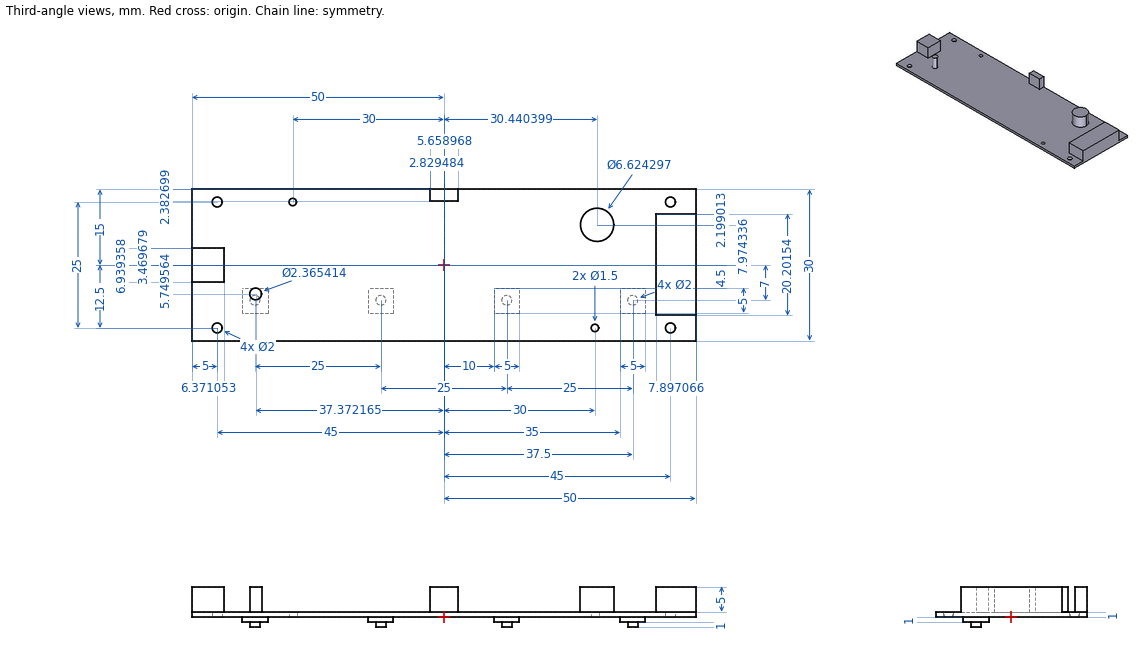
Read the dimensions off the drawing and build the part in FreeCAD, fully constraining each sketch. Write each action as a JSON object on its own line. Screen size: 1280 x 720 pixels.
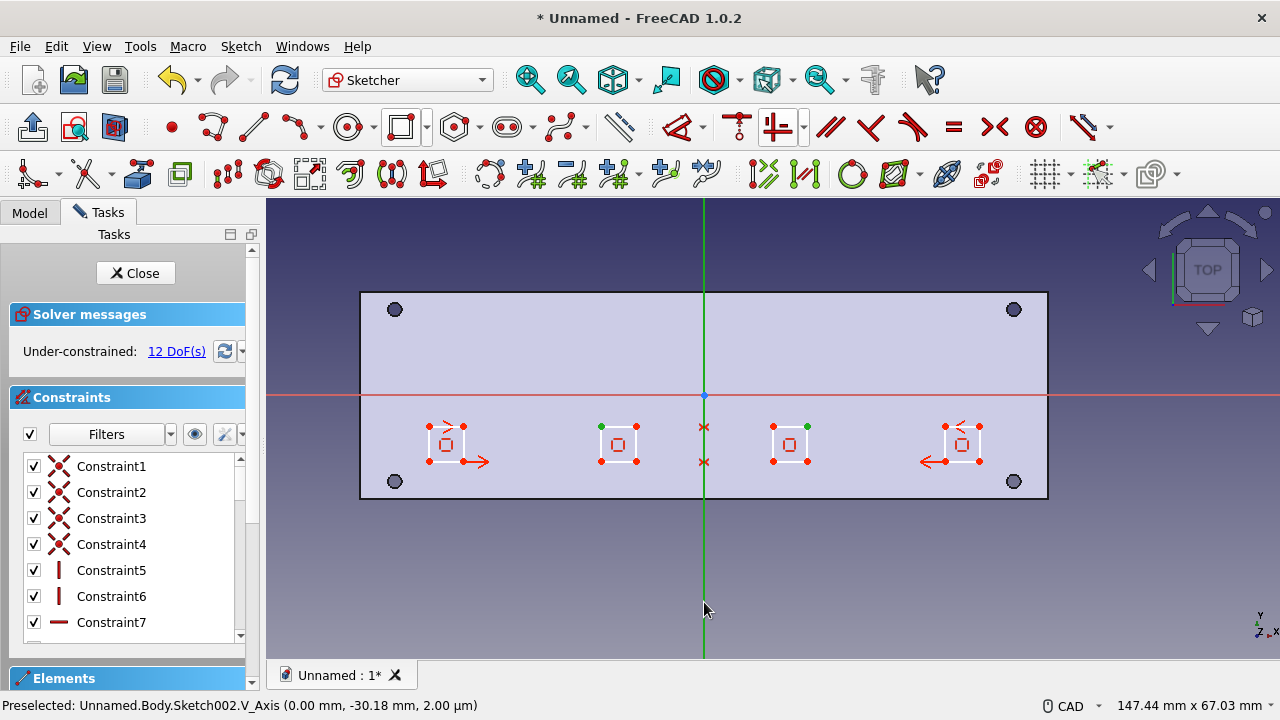
{"action": "key", "text": "s"}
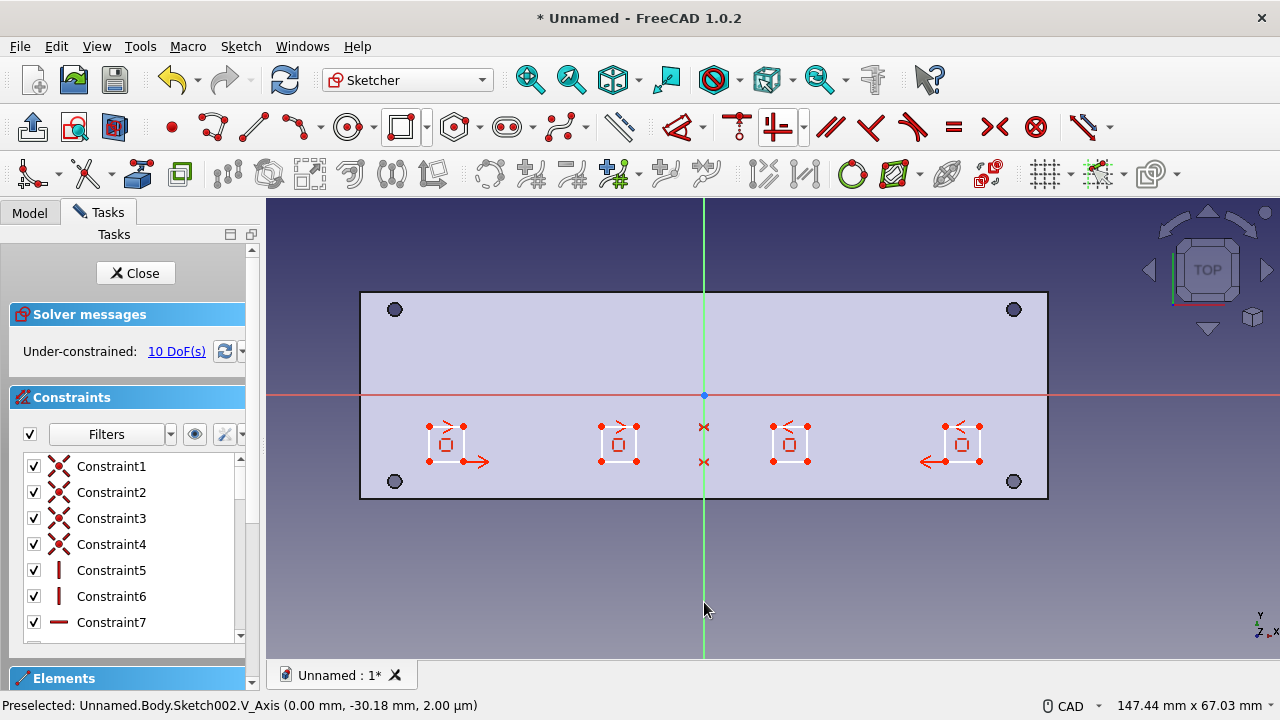
{"action": "left_click", "coordinate": [773, 462]}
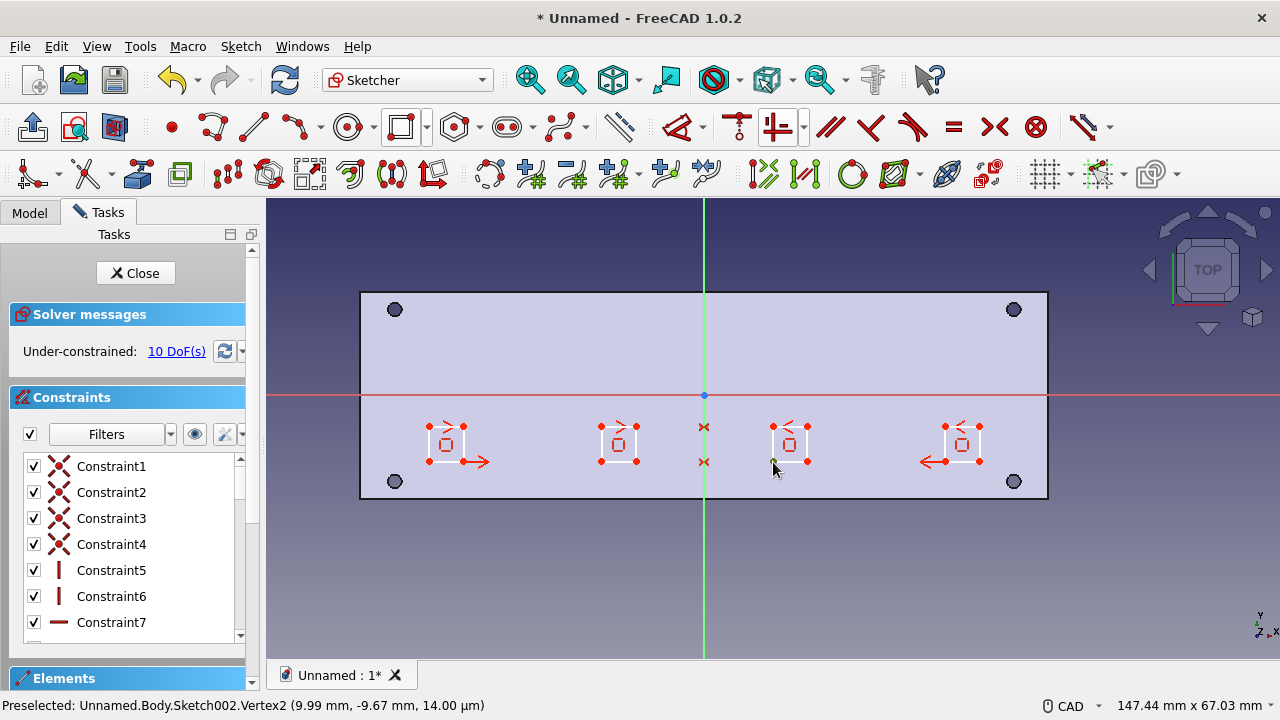
{"action": "left_click", "coordinate": [636, 462]}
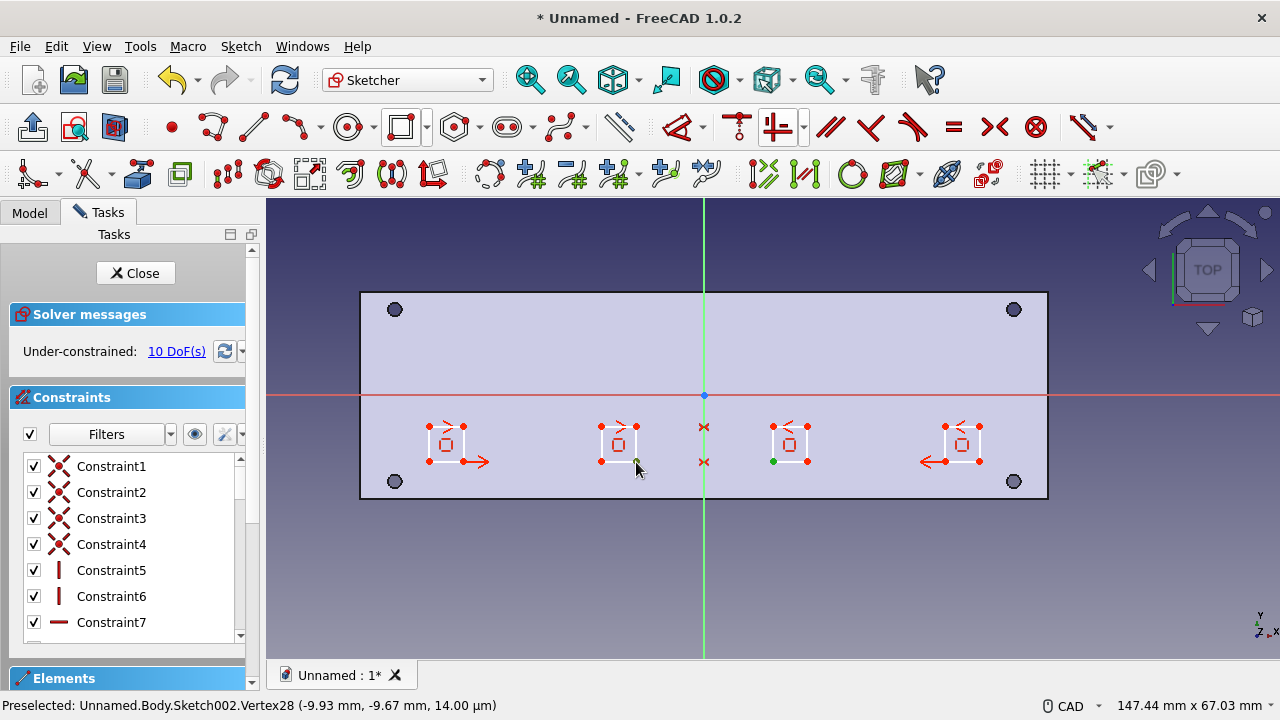
{"action": "left_click", "coordinate": [704, 602]}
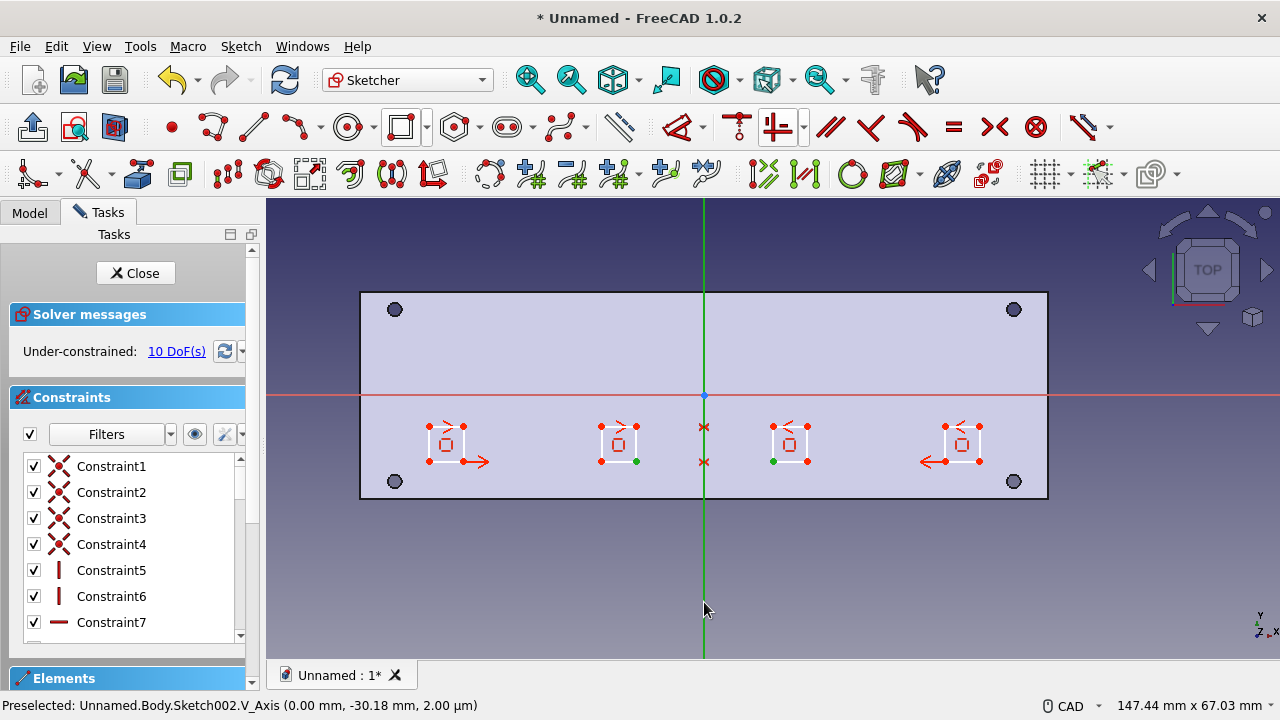
{"action": "key", "text": "s"}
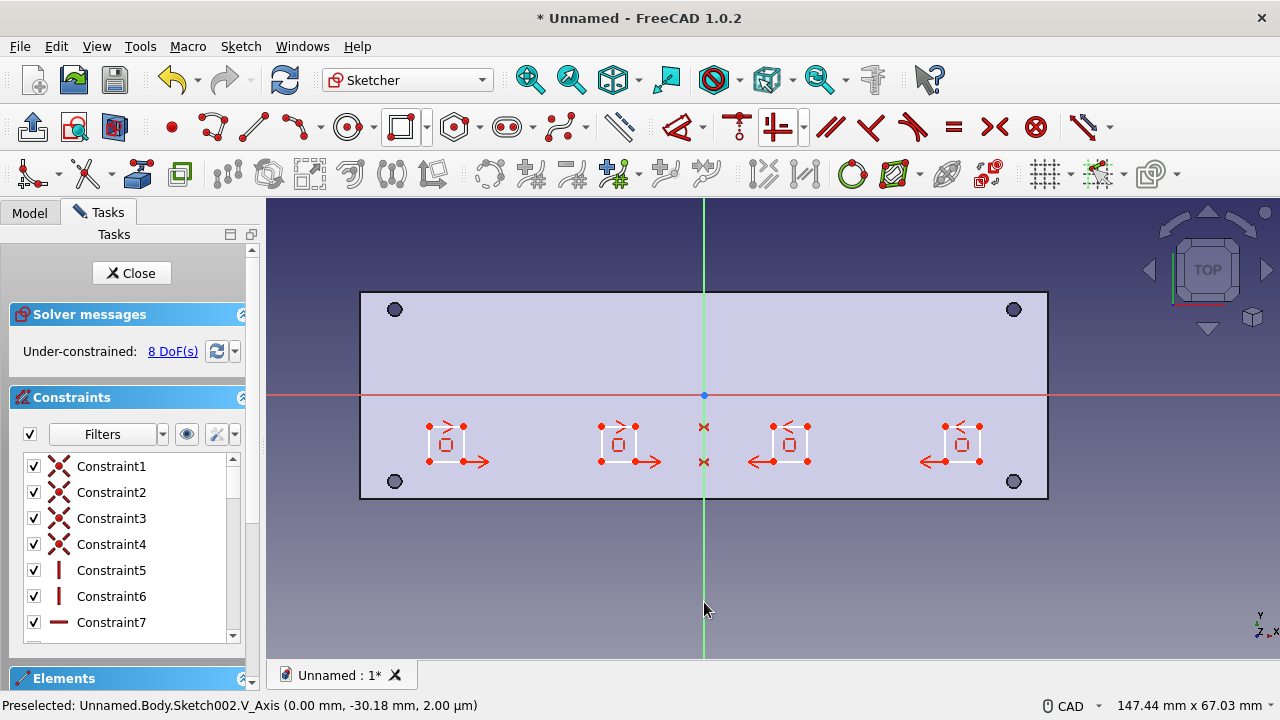
{"action": "left_click", "coordinate": [676, 128]}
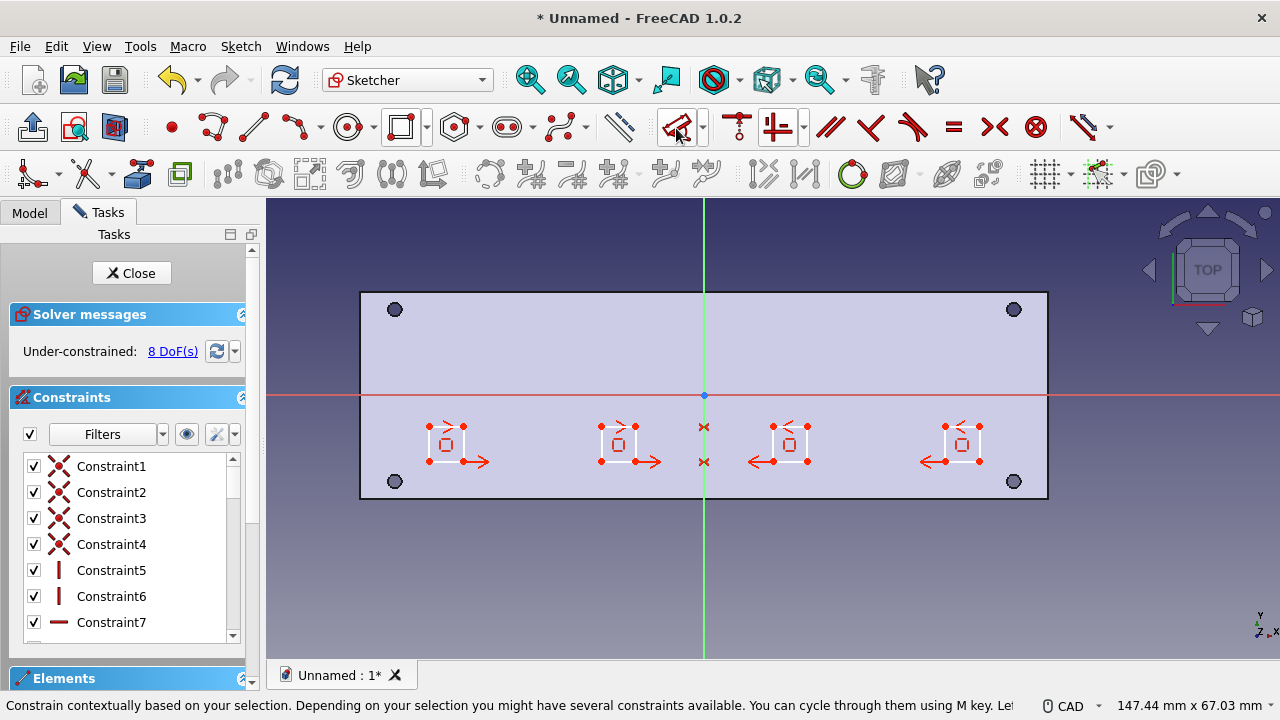
{"action": "scroll", "coordinate": [773, 437], "scroll_direction": "up", "scroll_amount": 2}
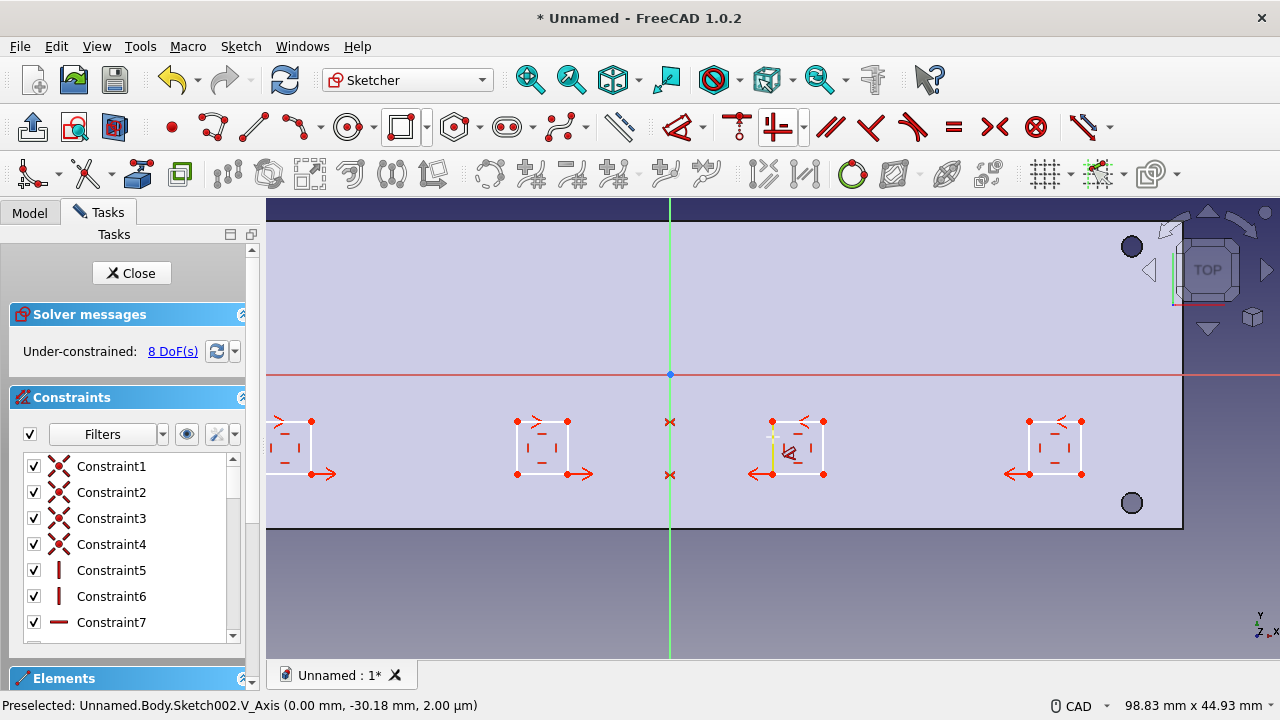
{"action": "left_click", "coordinate": [773, 437]}
{"action": "left_click", "coordinate": [807, 448]}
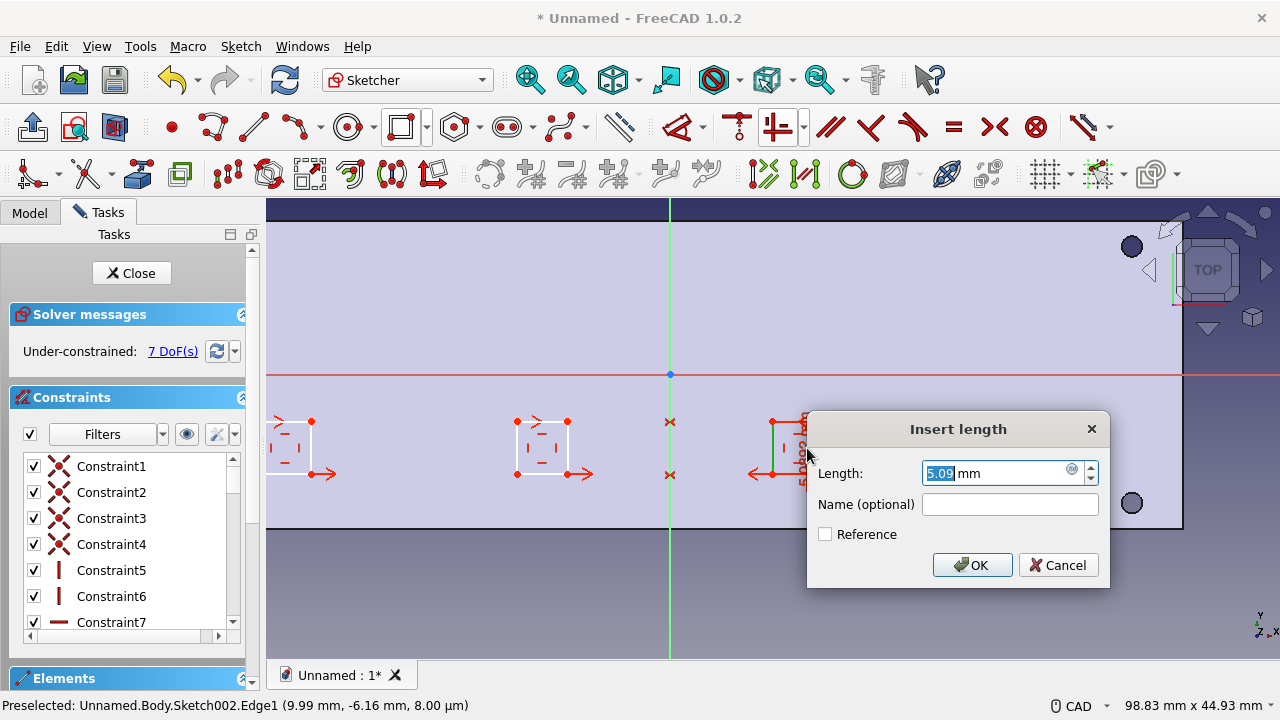
{"action": "type", "text": "5"}
{"action": "key", "text": "Return"}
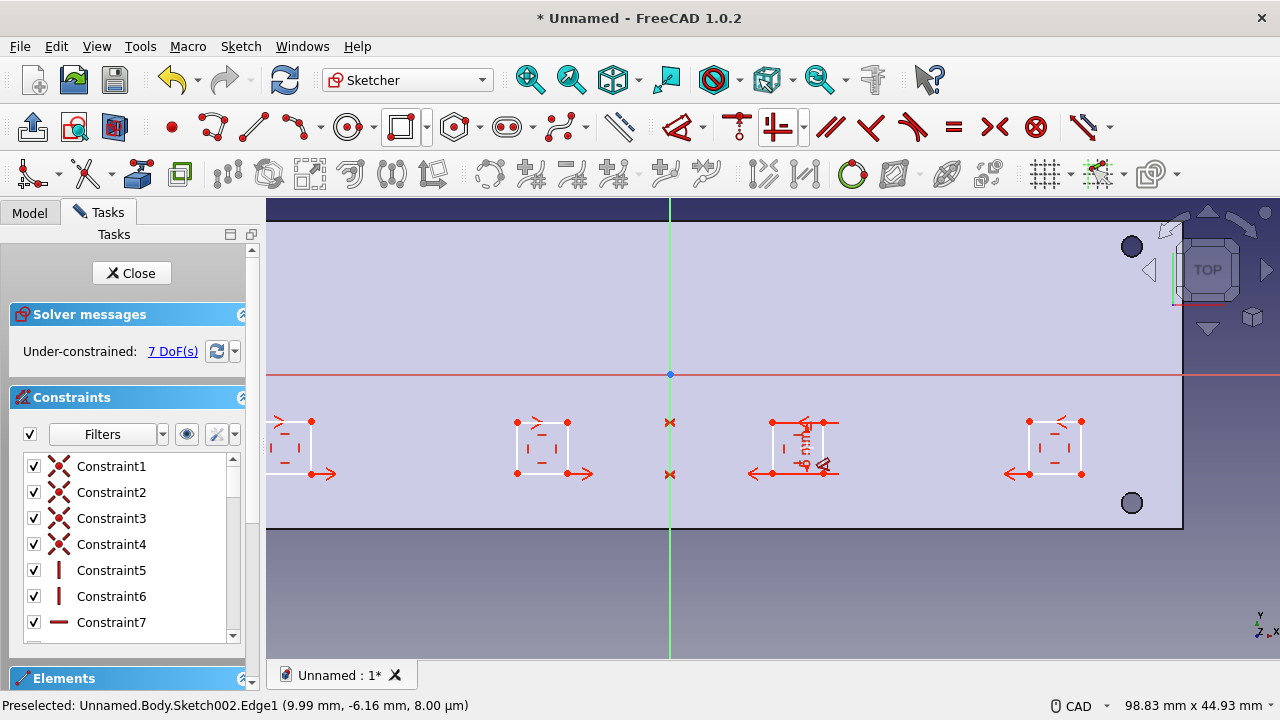
{"action": "left_click", "coordinate": [788, 474]}
{"action": "left_click", "coordinate": [798, 508]}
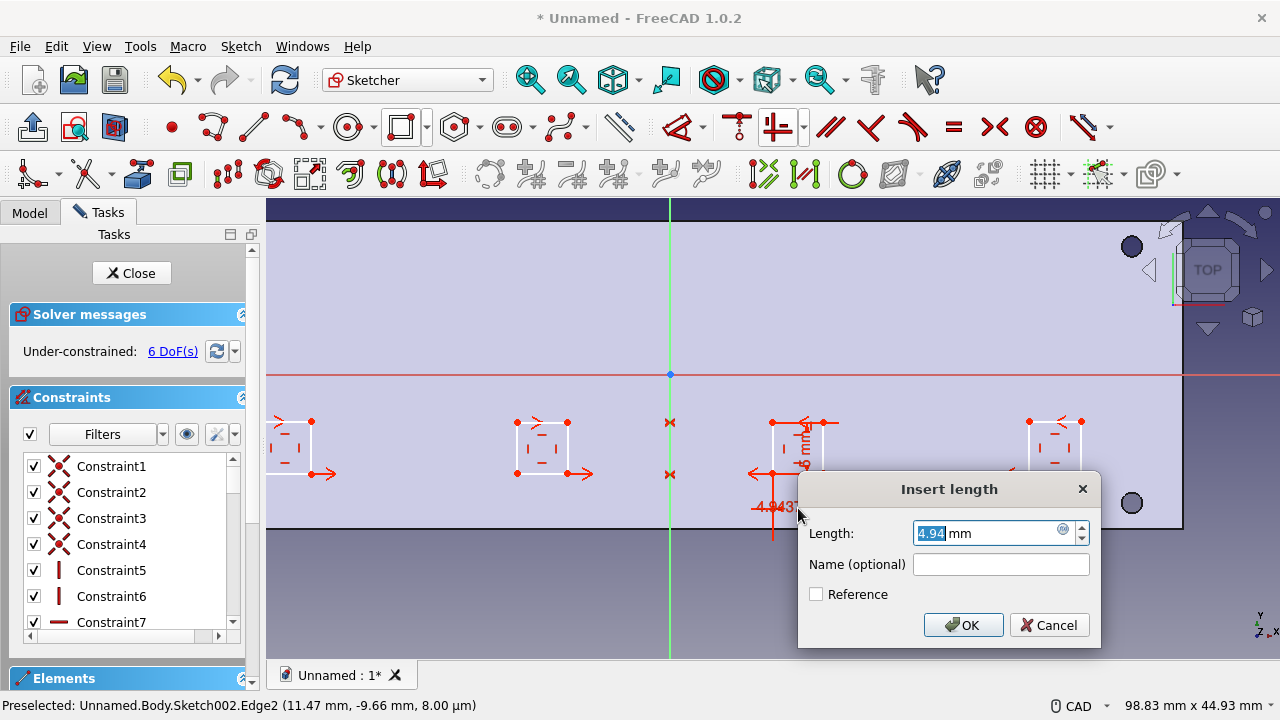
{"action": "type", "text": "5"}
{"action": "key", "text": "Return"}